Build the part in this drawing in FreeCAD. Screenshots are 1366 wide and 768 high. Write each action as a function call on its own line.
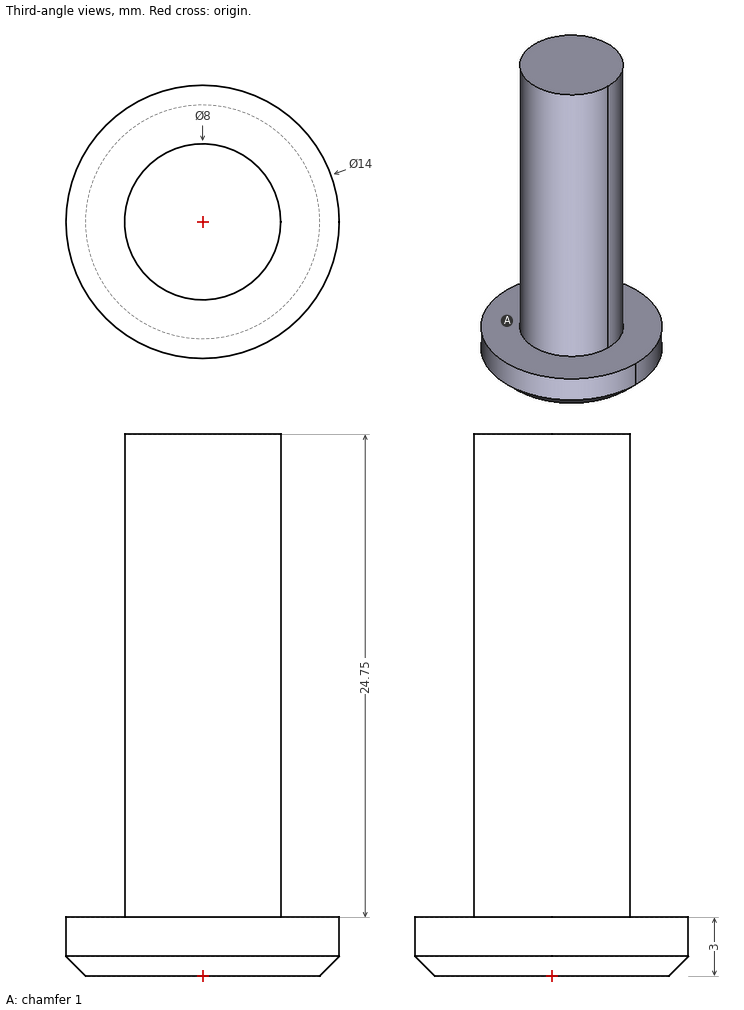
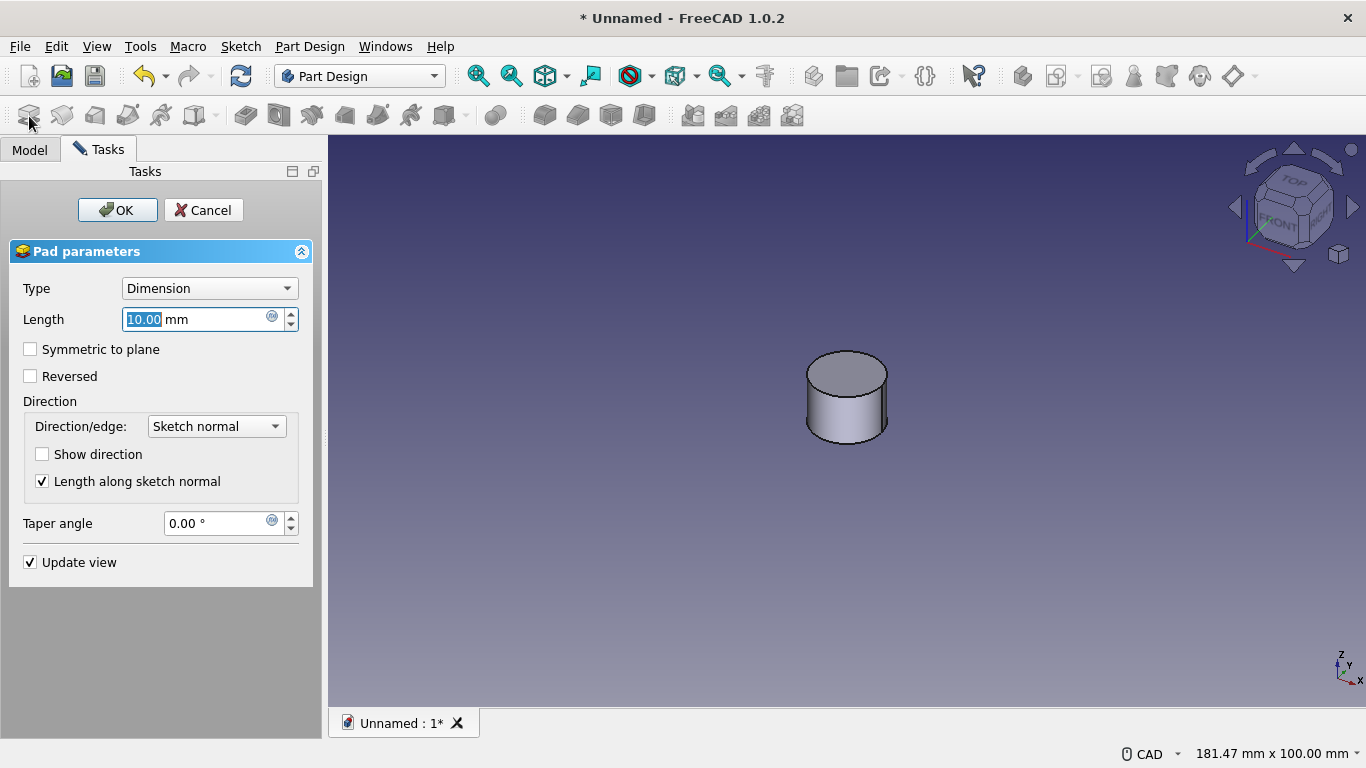
text(3)
key(Tab)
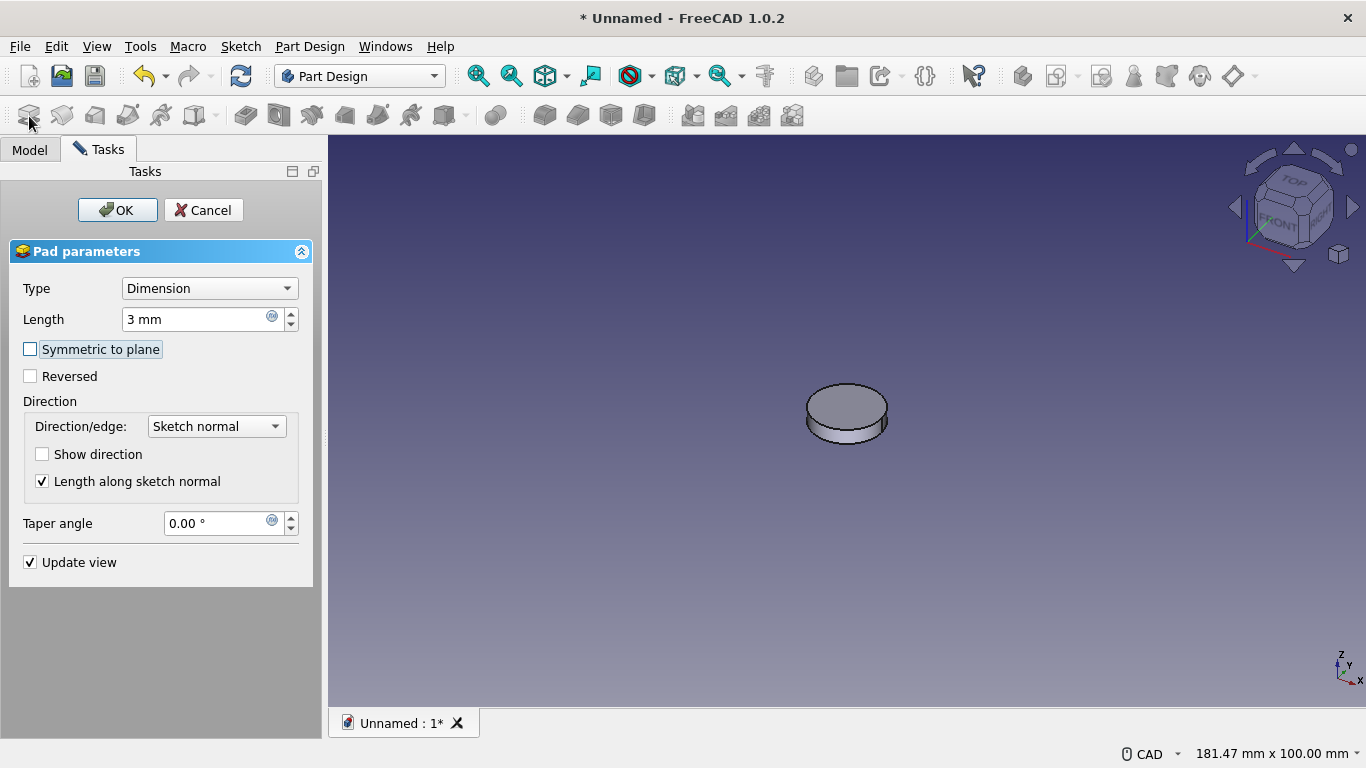
click(118, 210)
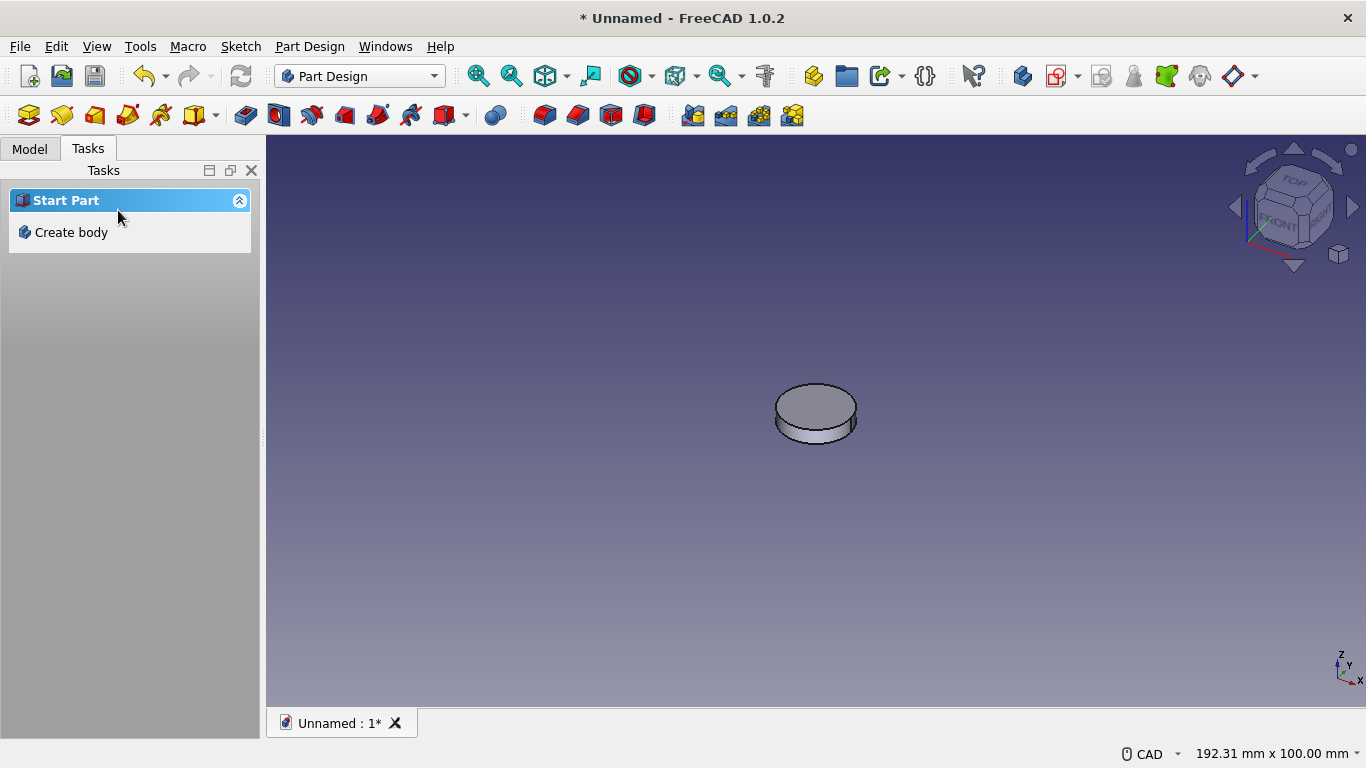
click(479, 76)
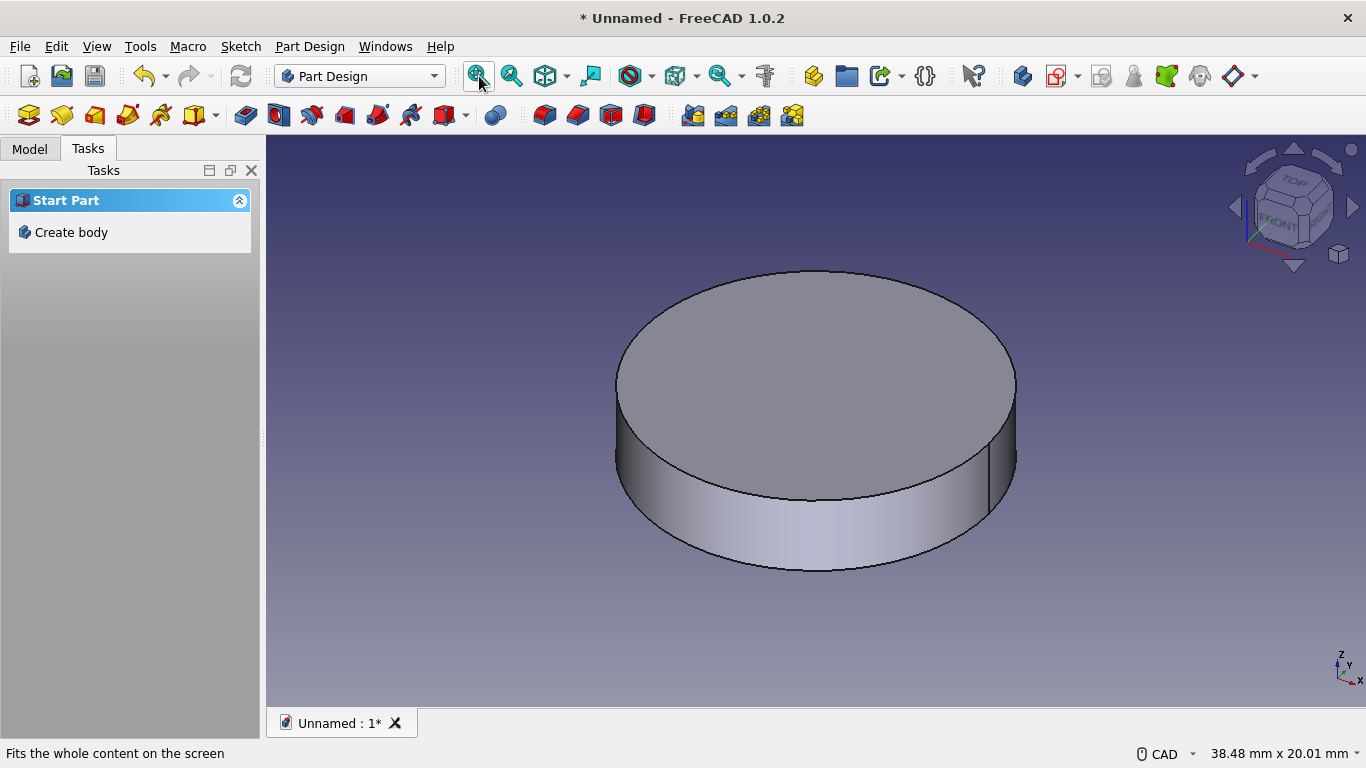
click(816, 385)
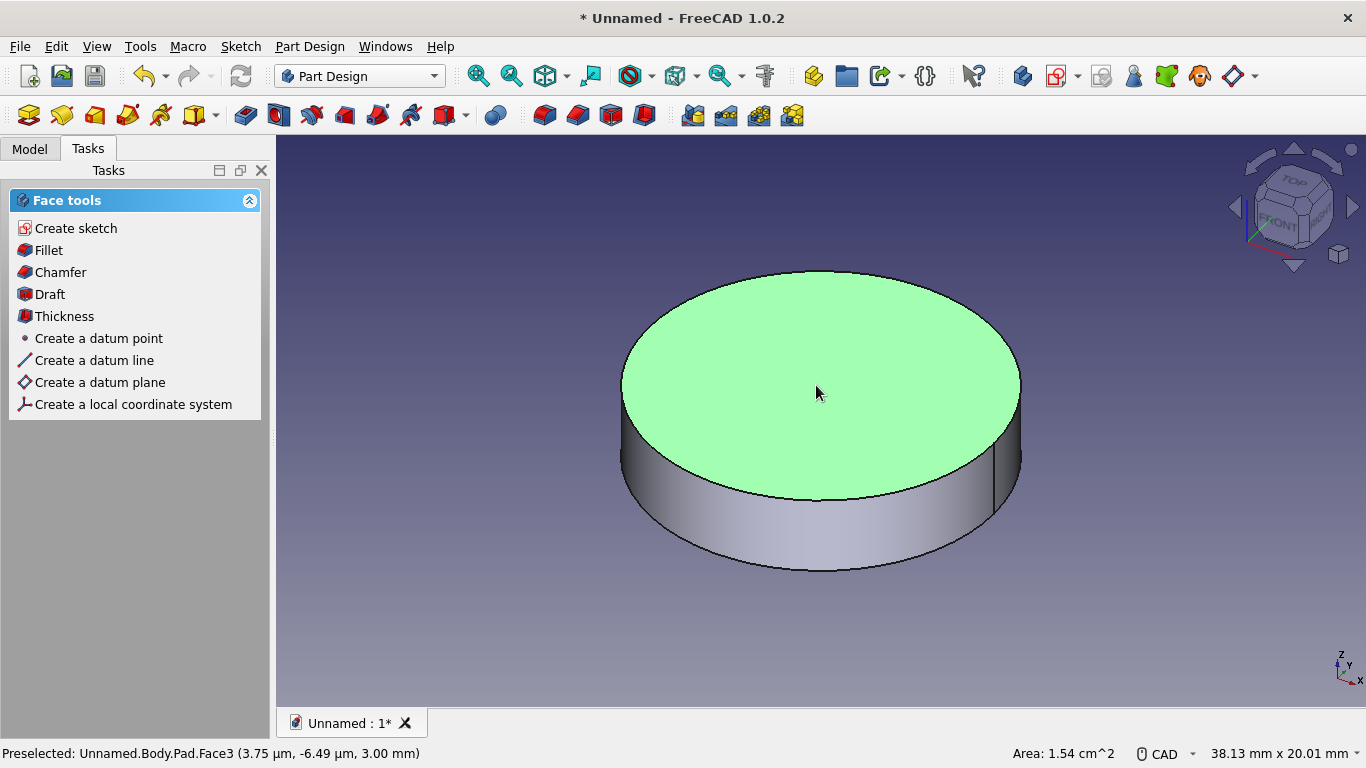
click(1056, 76)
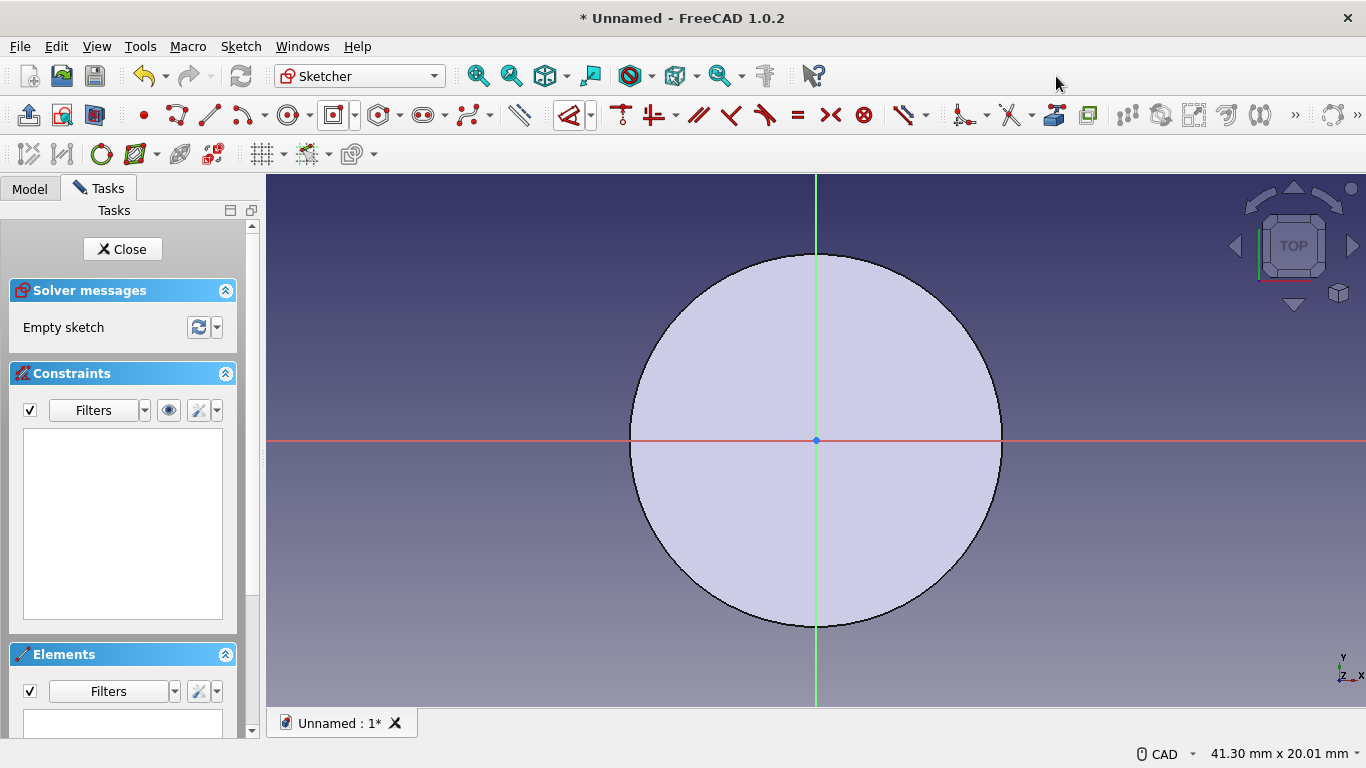
scroll(955, 440, up, 2)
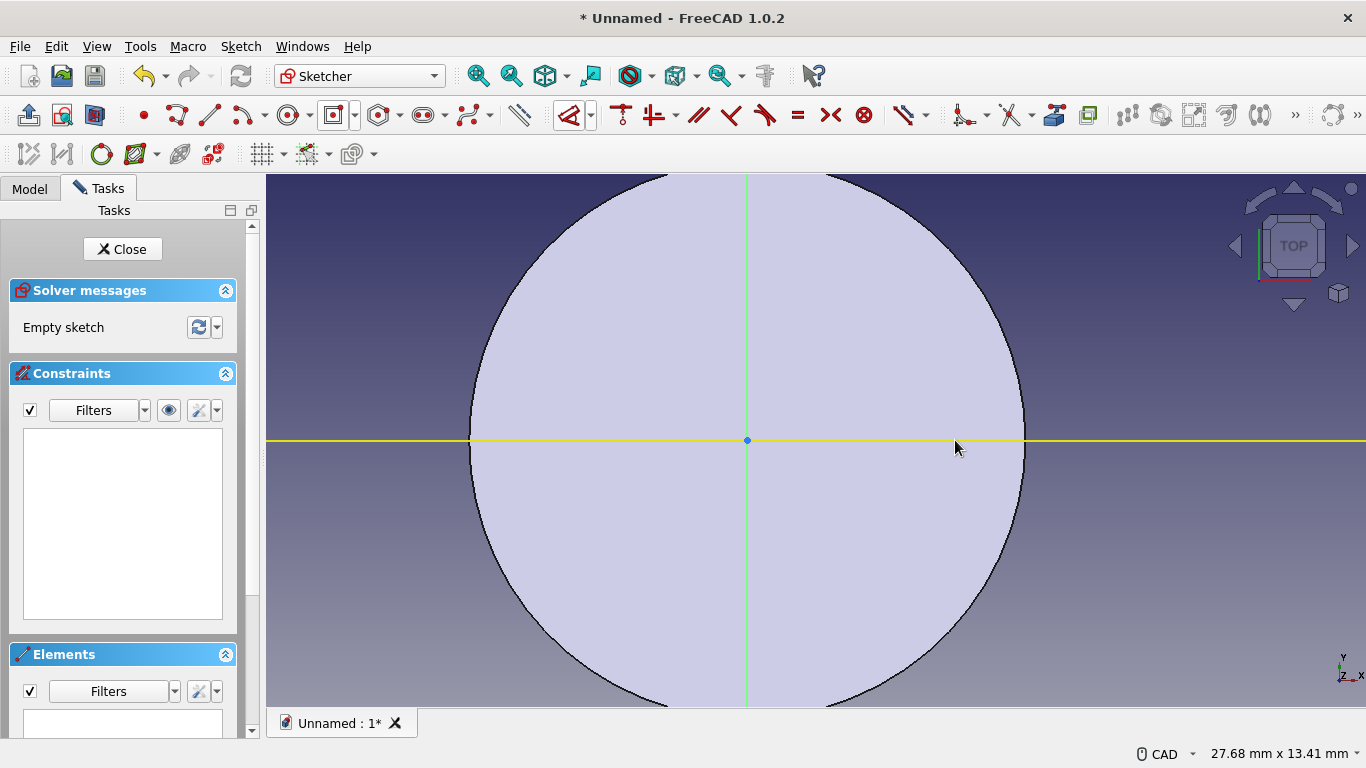
click(288, 116)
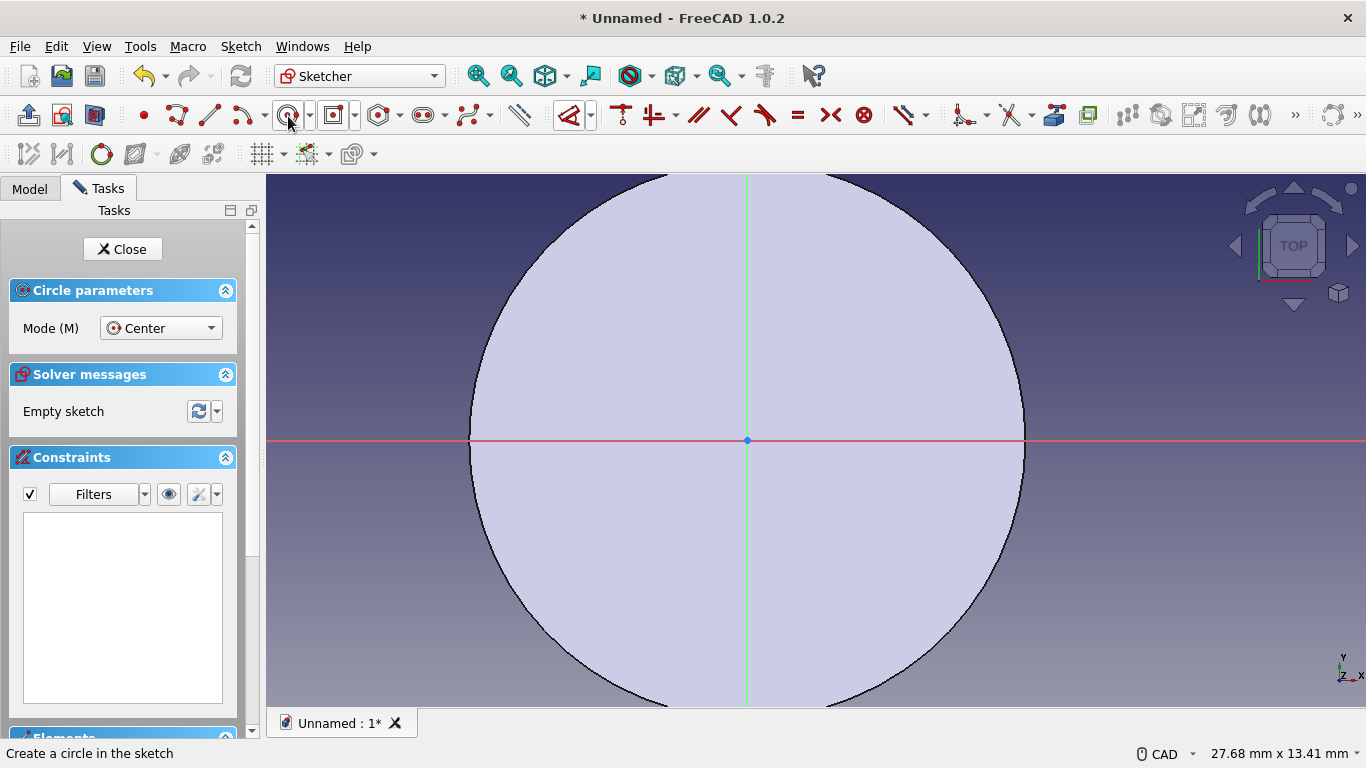
click(747, 440)
move(860, 328)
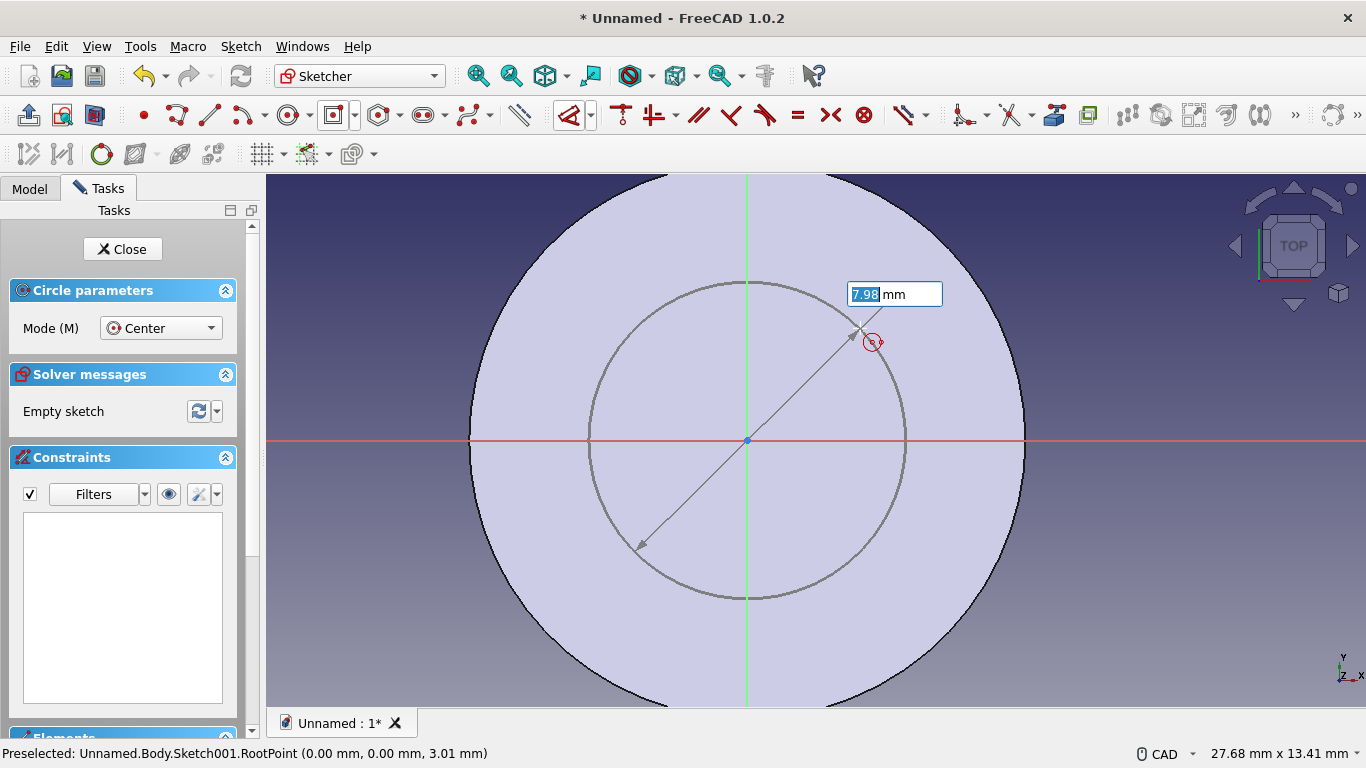
text(8)
key(Return)
key(Escape)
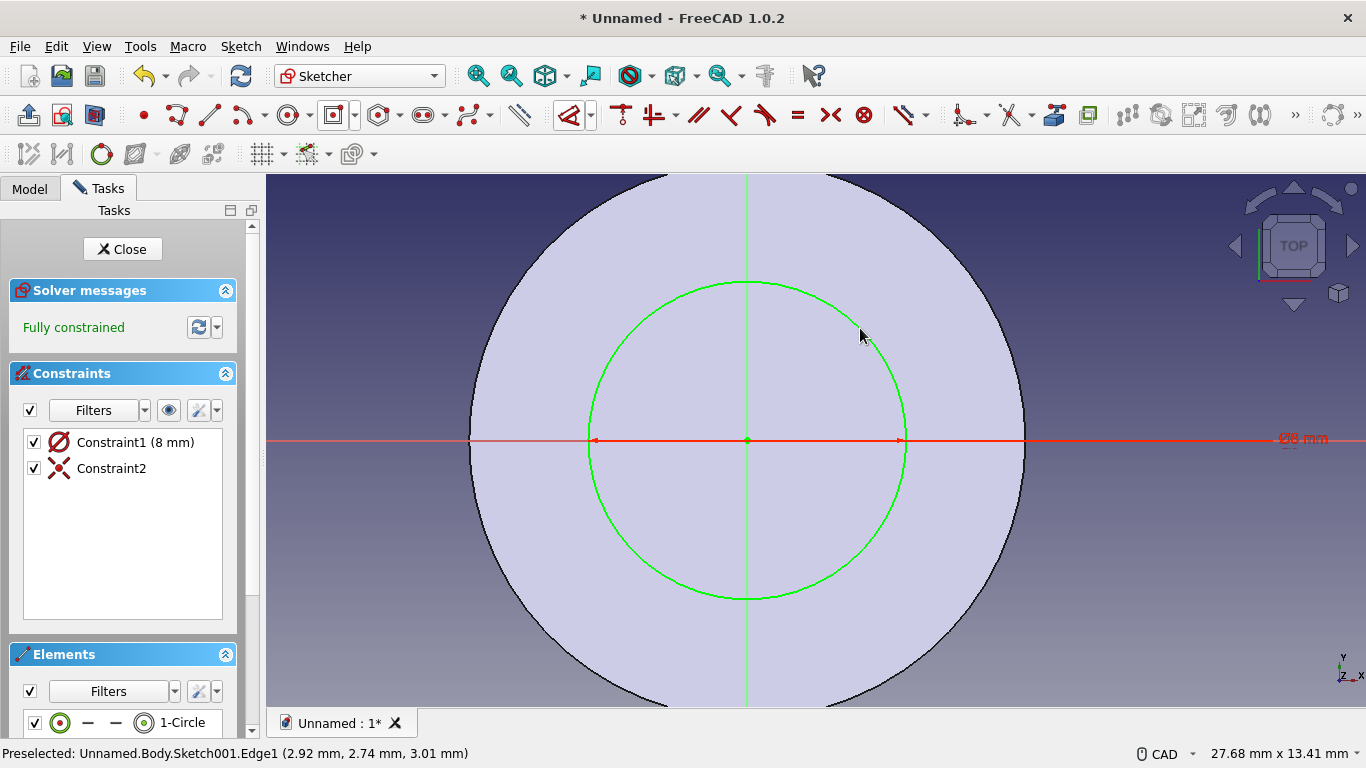
click(123, 249)